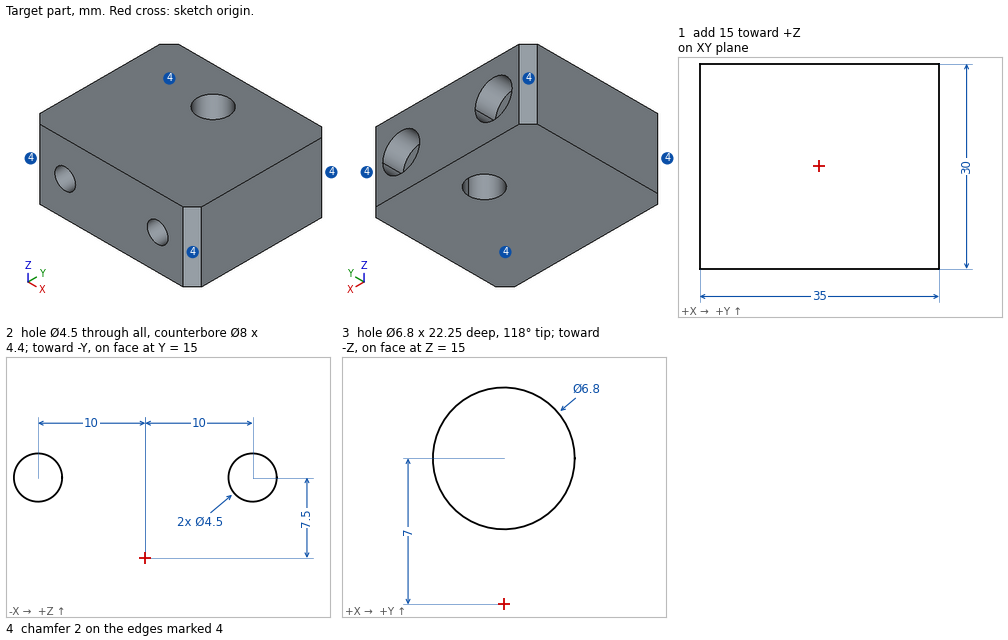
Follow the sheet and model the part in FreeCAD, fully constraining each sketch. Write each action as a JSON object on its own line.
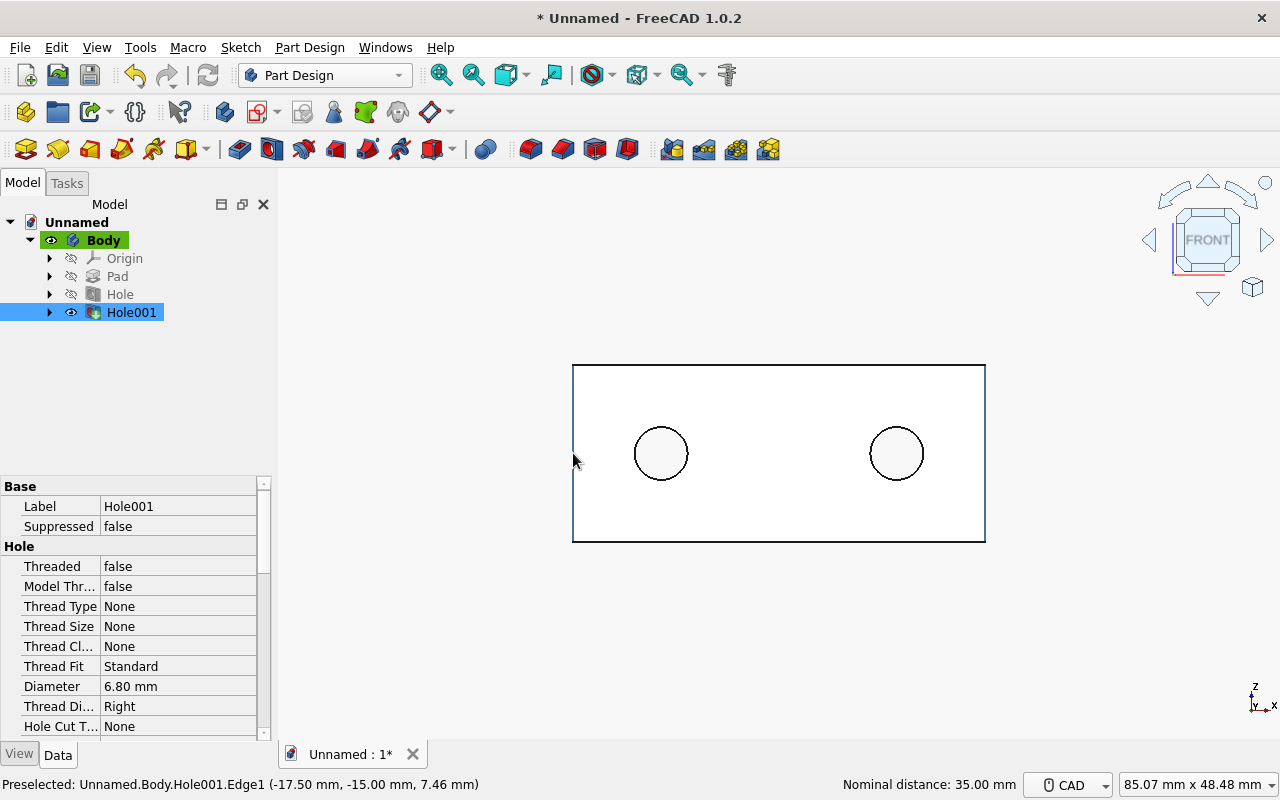
{"action": "key", "text": "3"}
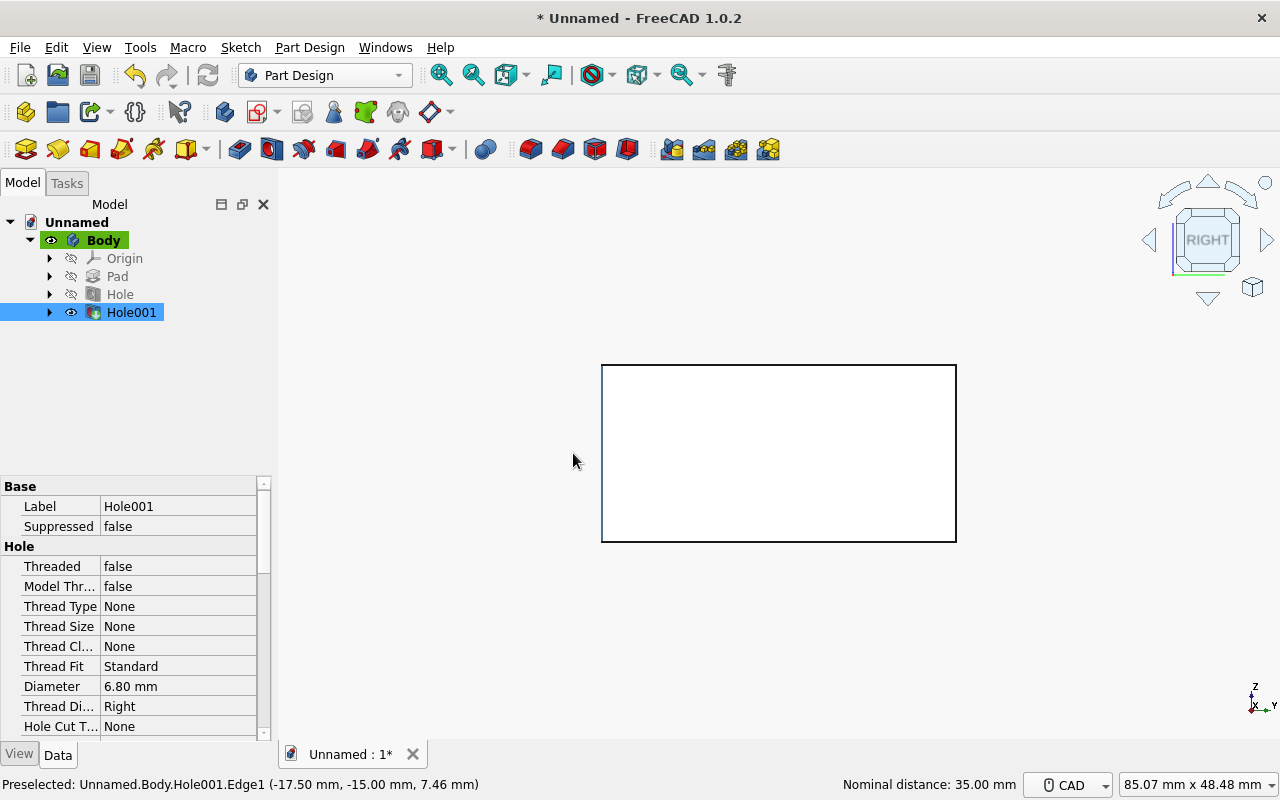
{"action": "left_click", "coordinate": [442, 76]}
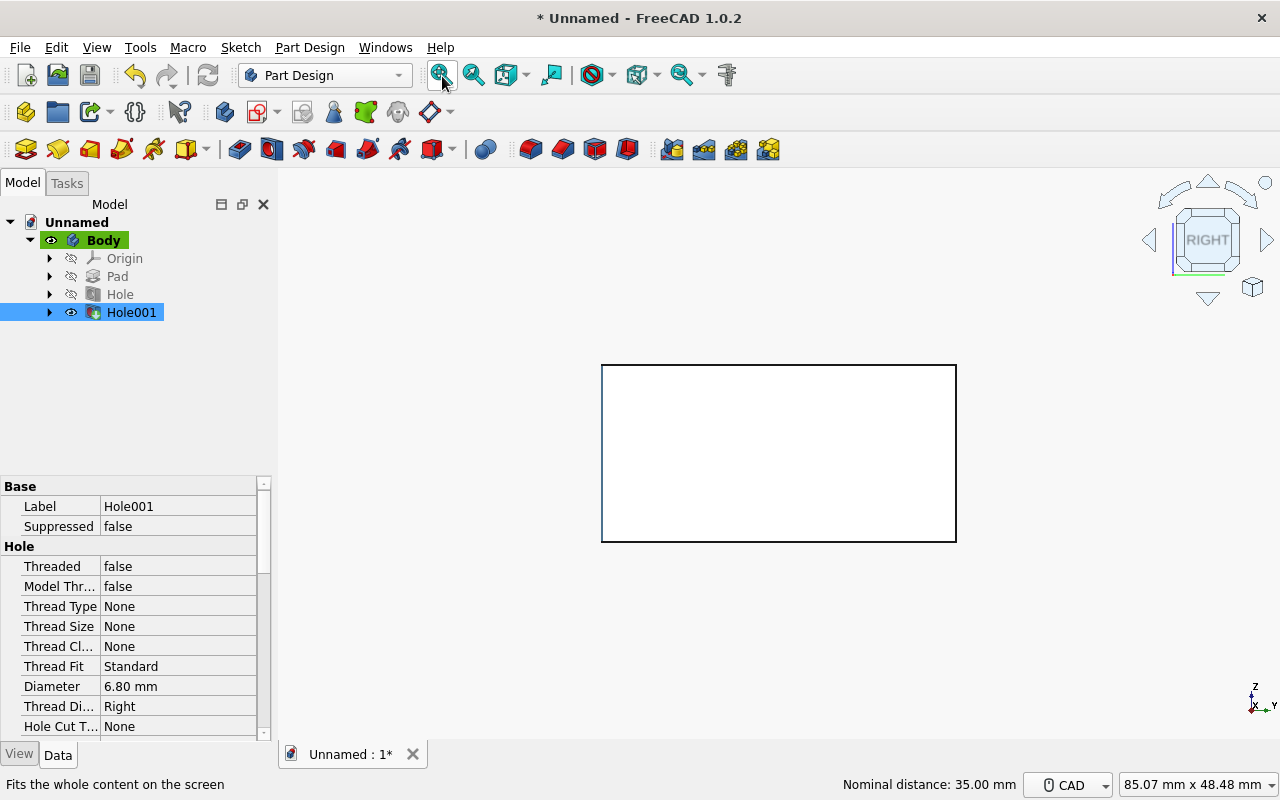
{"action": "left_click", "coordinate": [956, 452], "text": "ctrl"}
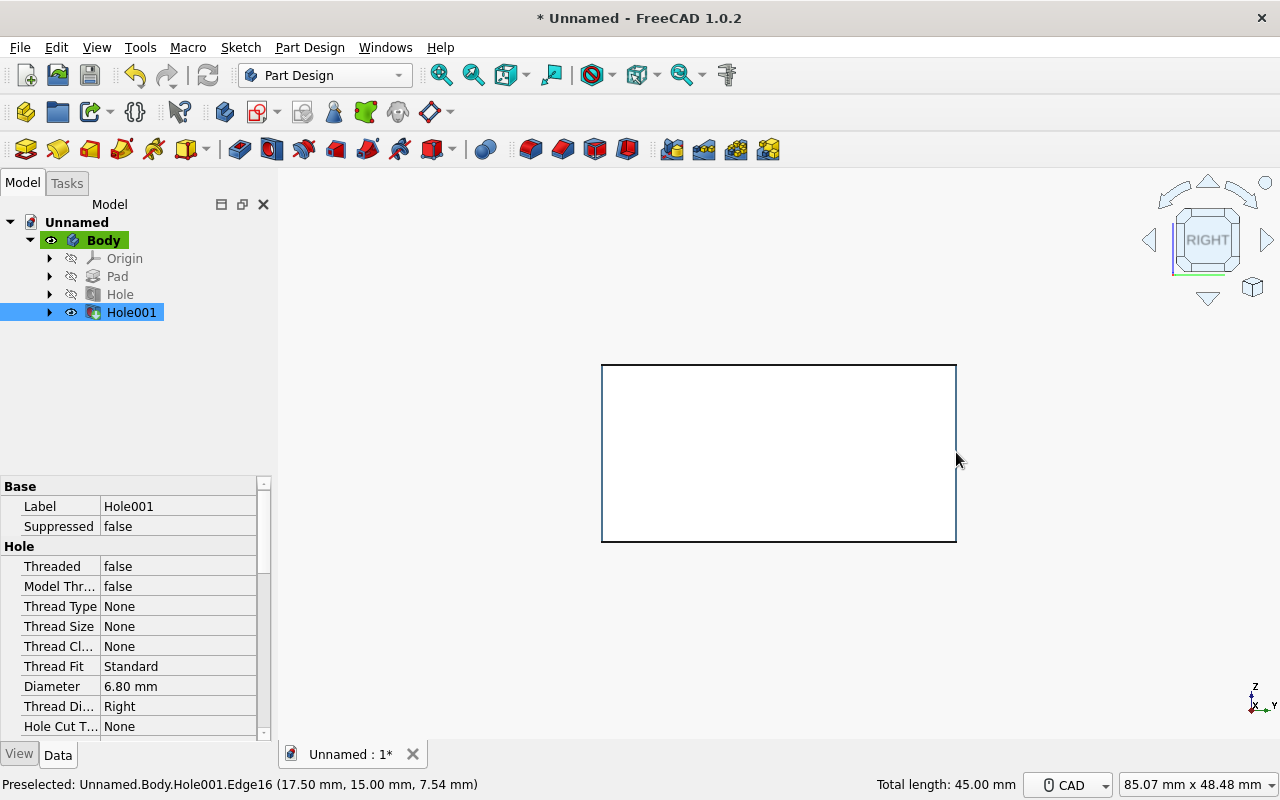
{"action": "key", "text": "5"}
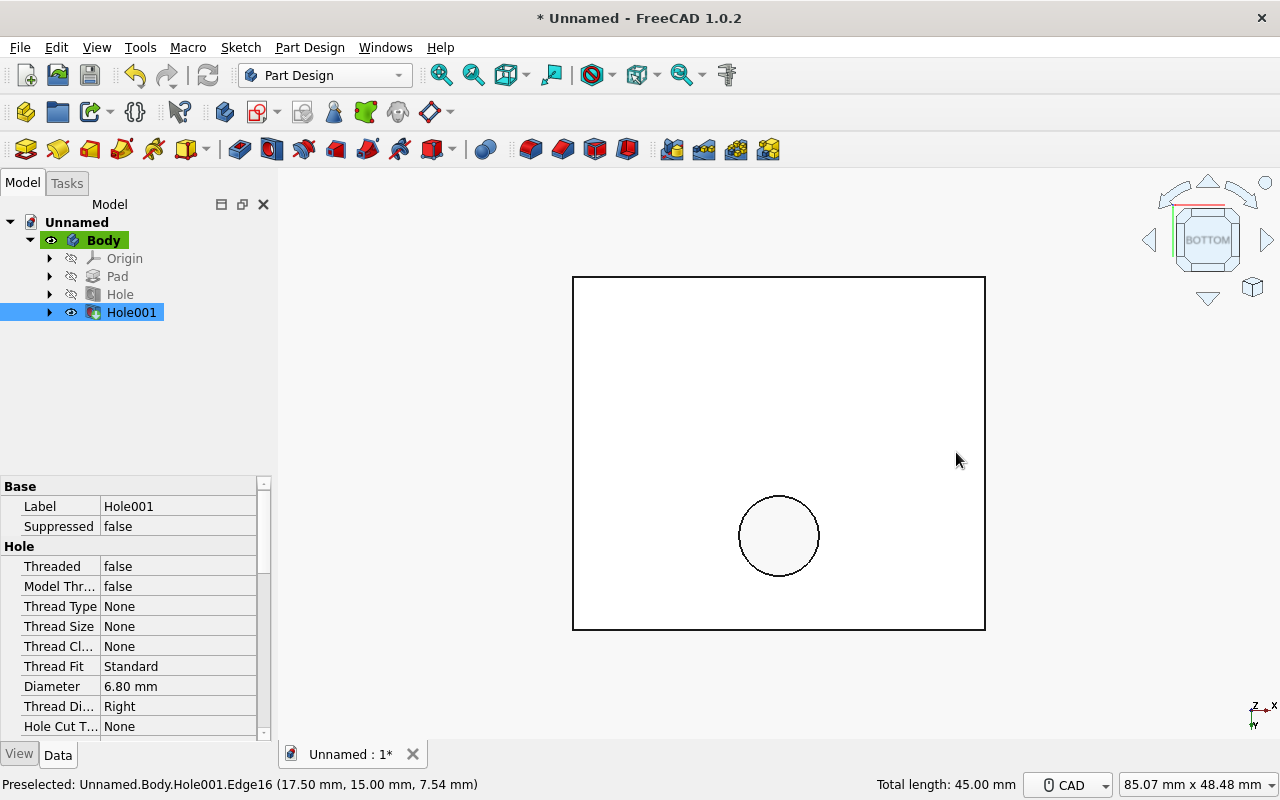
{"action": "key", "text": "4"}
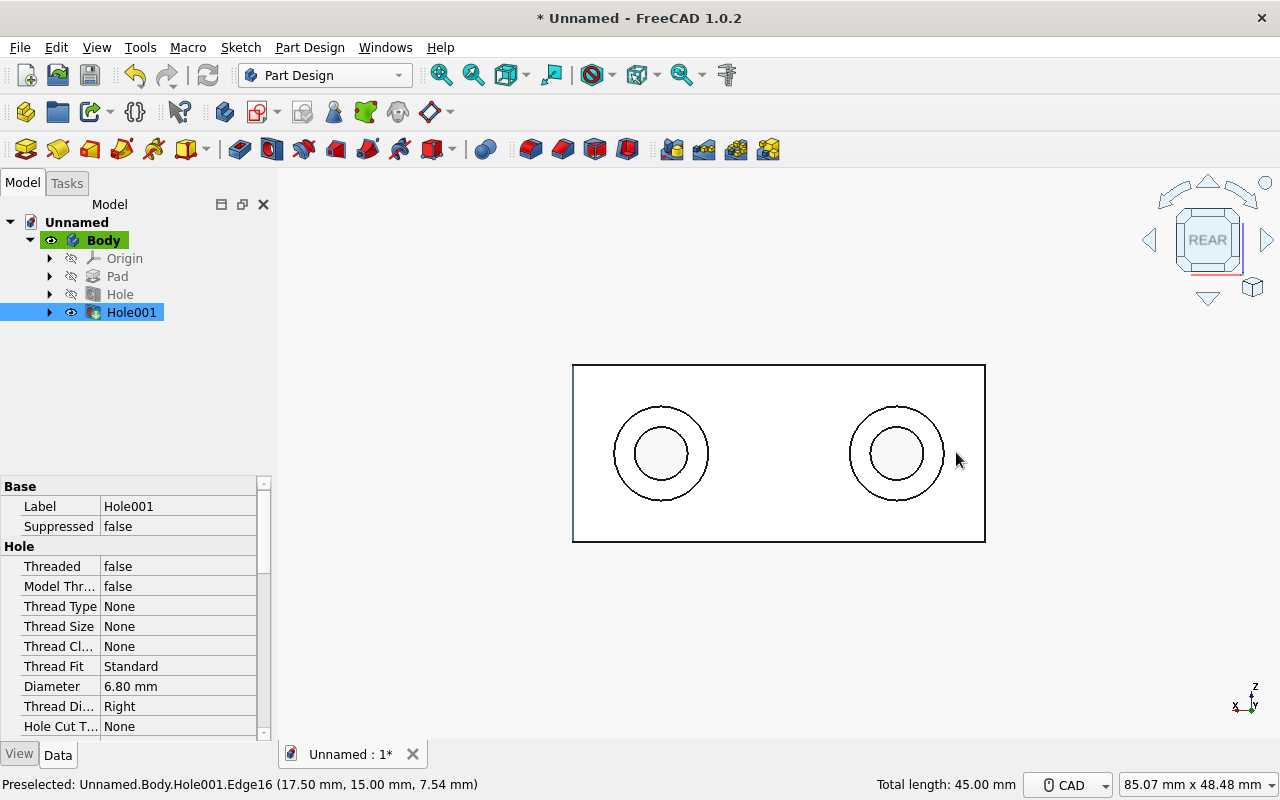
{"action": "key", "text": "v f"}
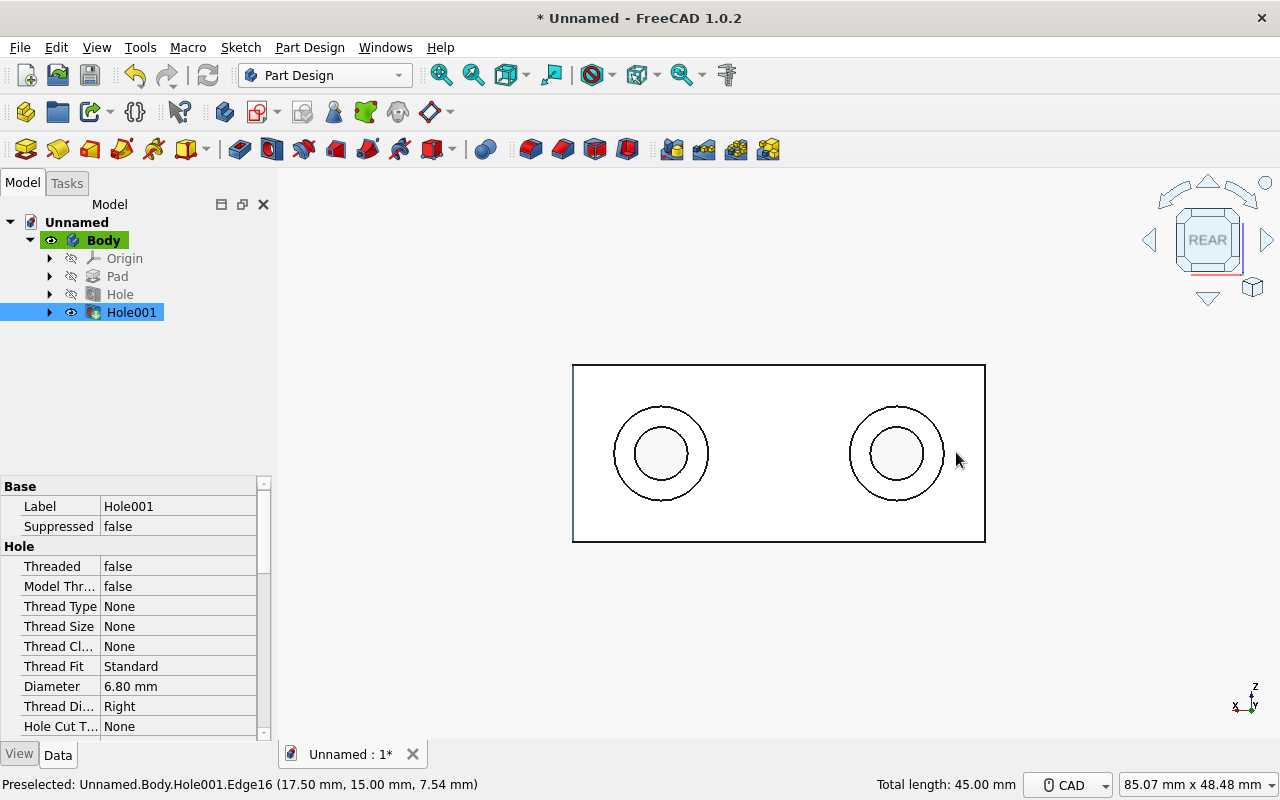
{"action": "left_click", "coordinate": [985, 453], "text": "ctrl"}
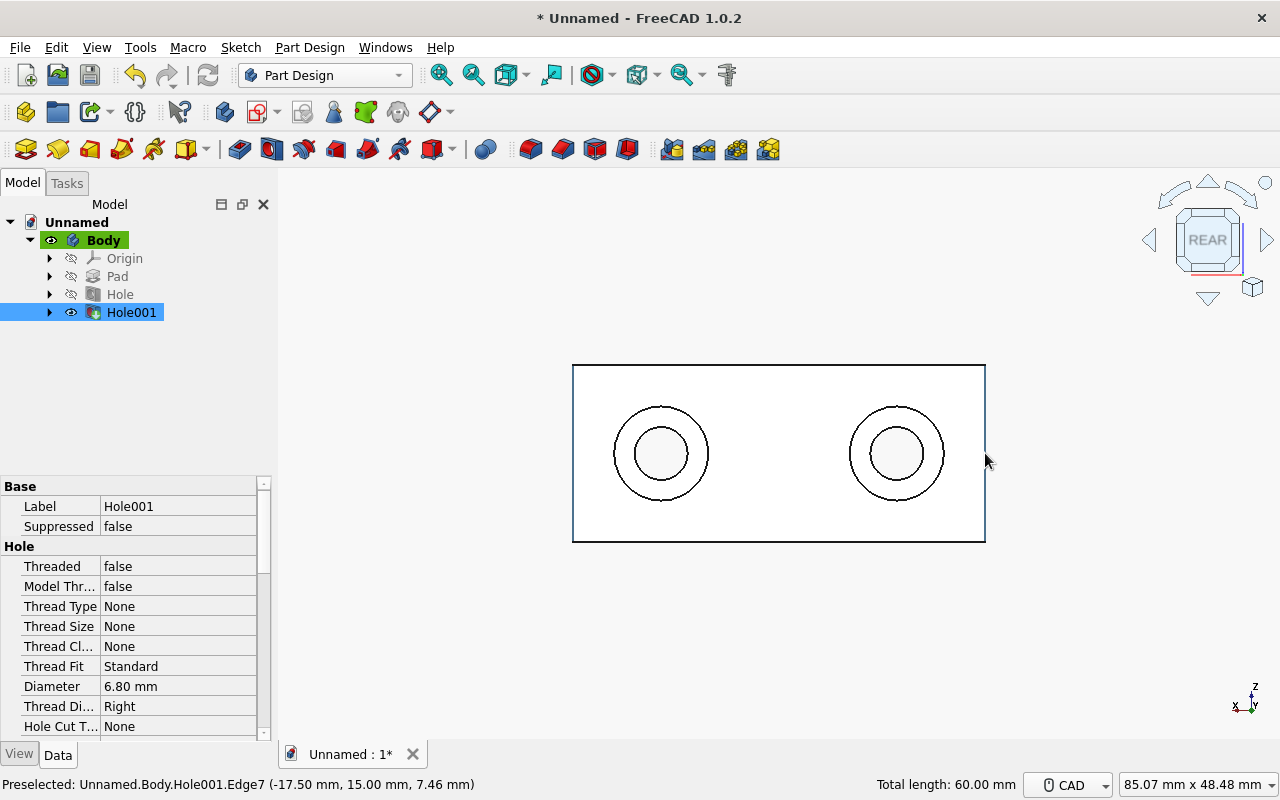
{"action": "left_click", "coordinate": [564, 150]}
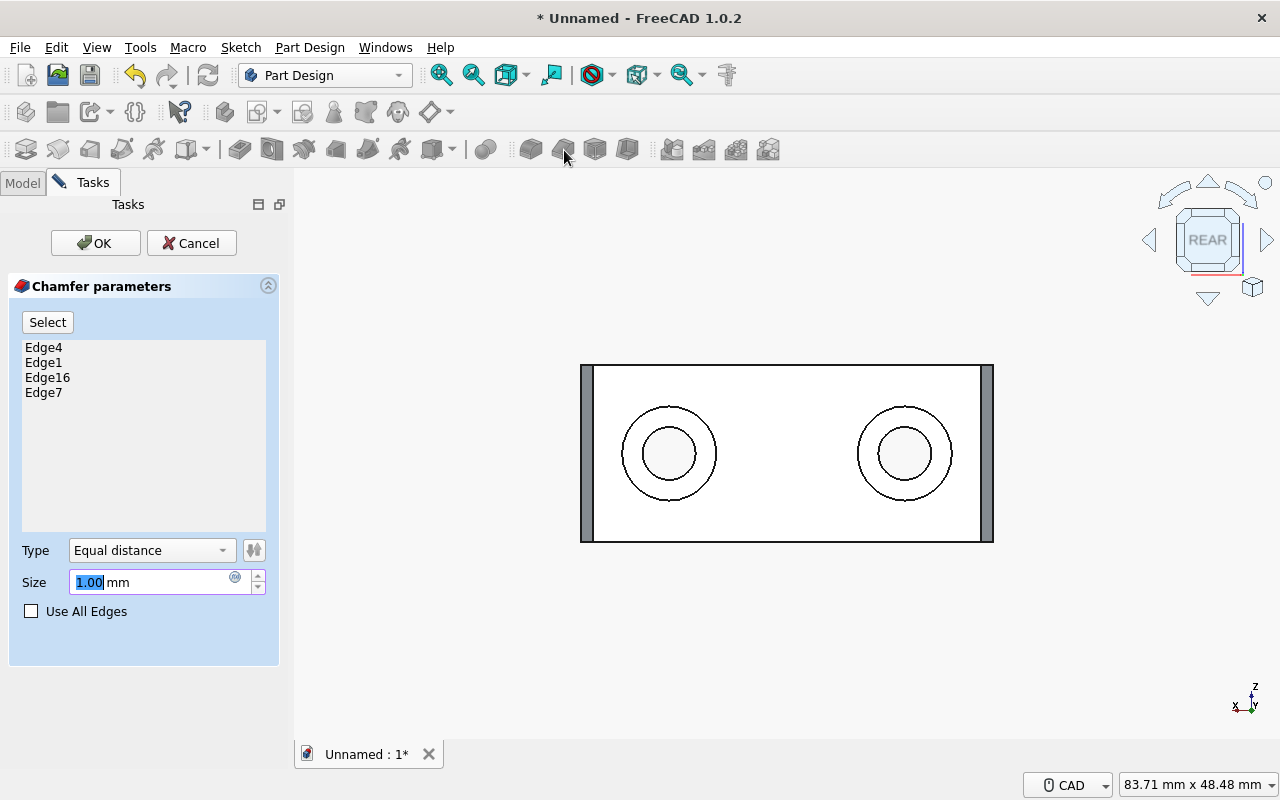
{"action": "type", "text": "2"}
{"action": "key", "text": "Tab"}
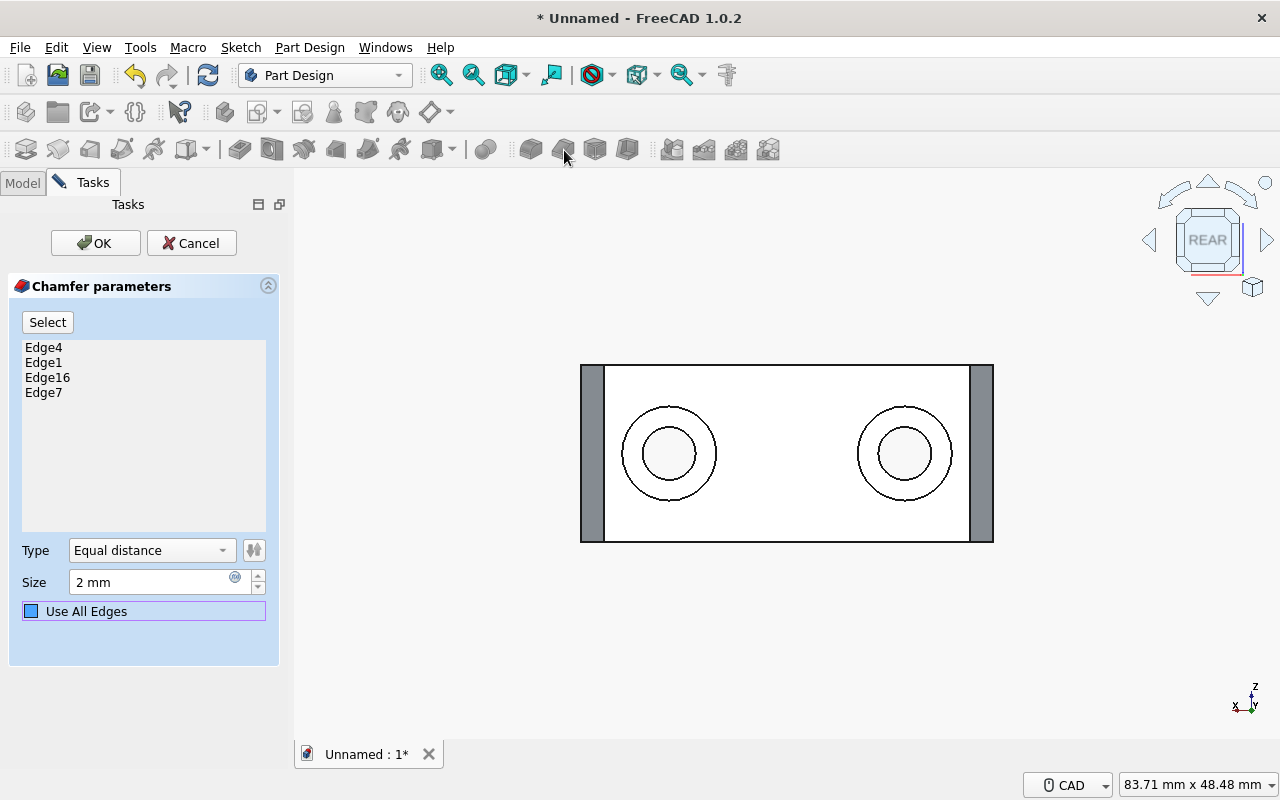
{"action": "left_click", "coordinate": [96, 243]}